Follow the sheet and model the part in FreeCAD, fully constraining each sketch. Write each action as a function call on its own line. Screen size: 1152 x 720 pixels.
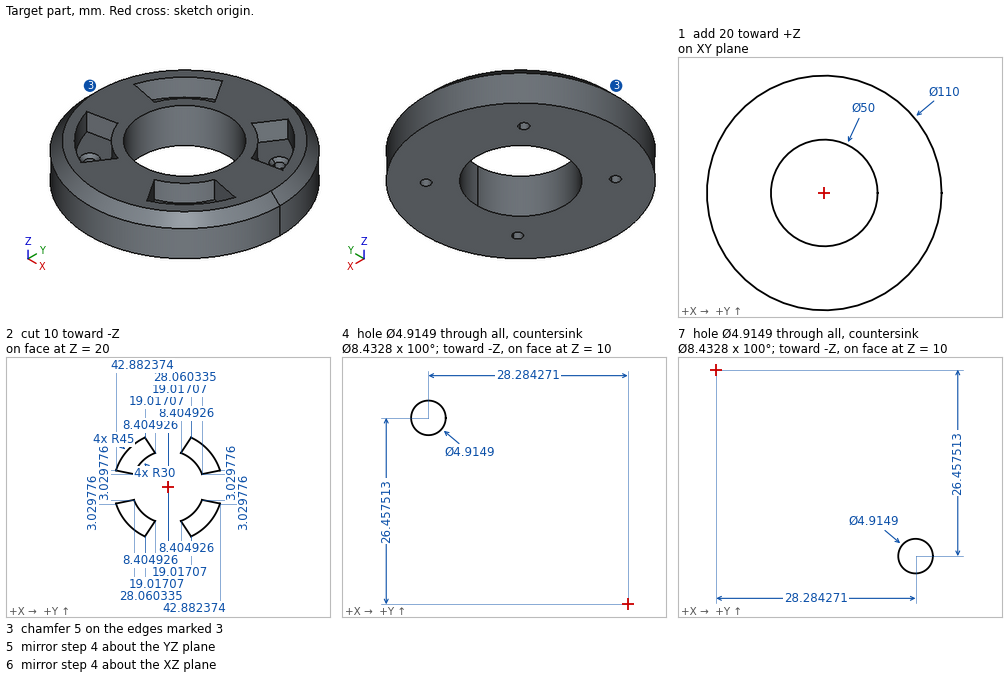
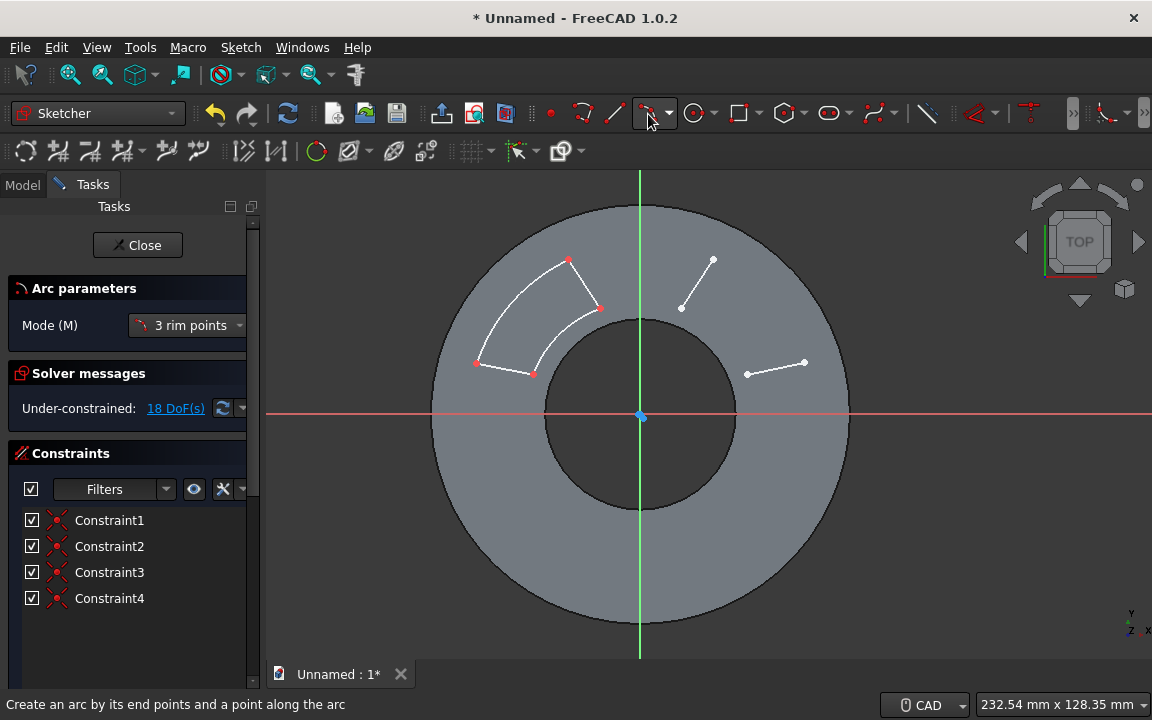
click(804, 363)
click(713, 260)
click(769, 301)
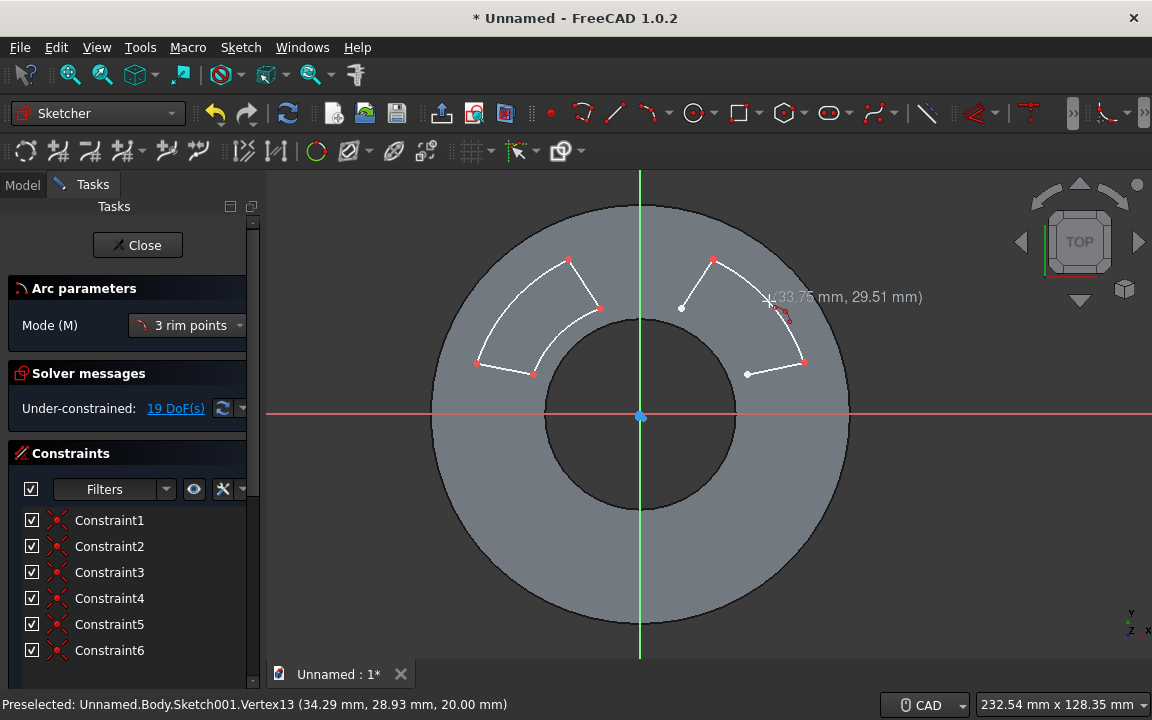
click(681, 309)
click(747, 375)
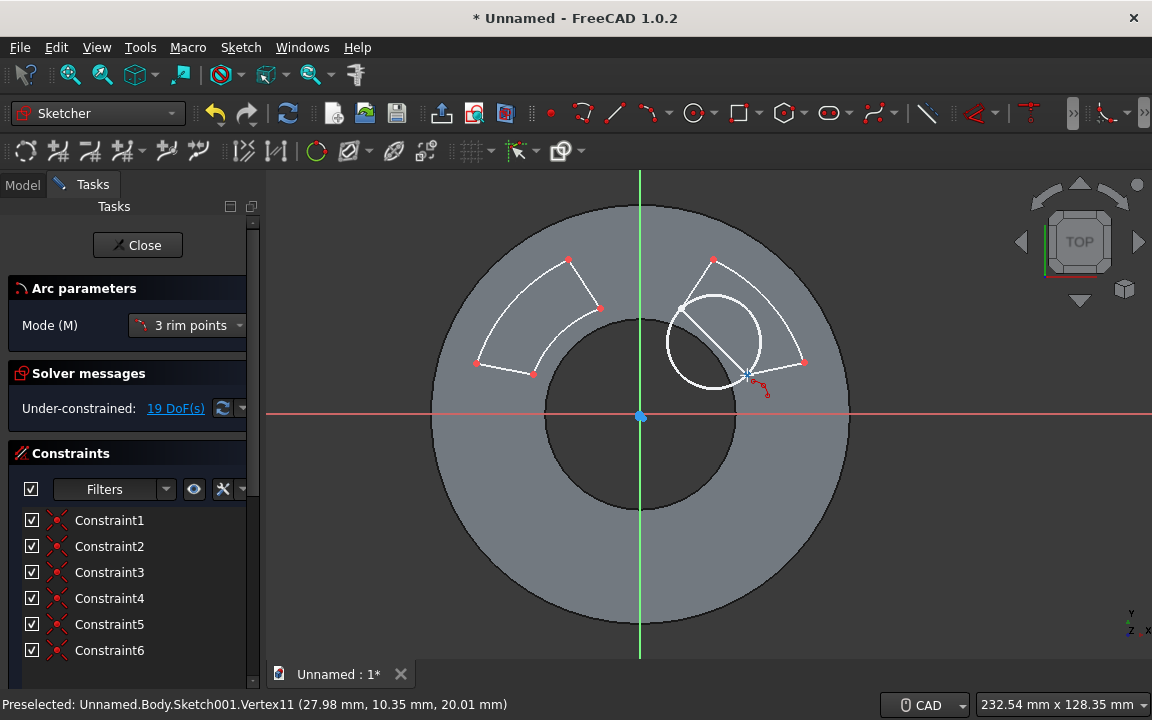
scroll(721, 334, up, 3)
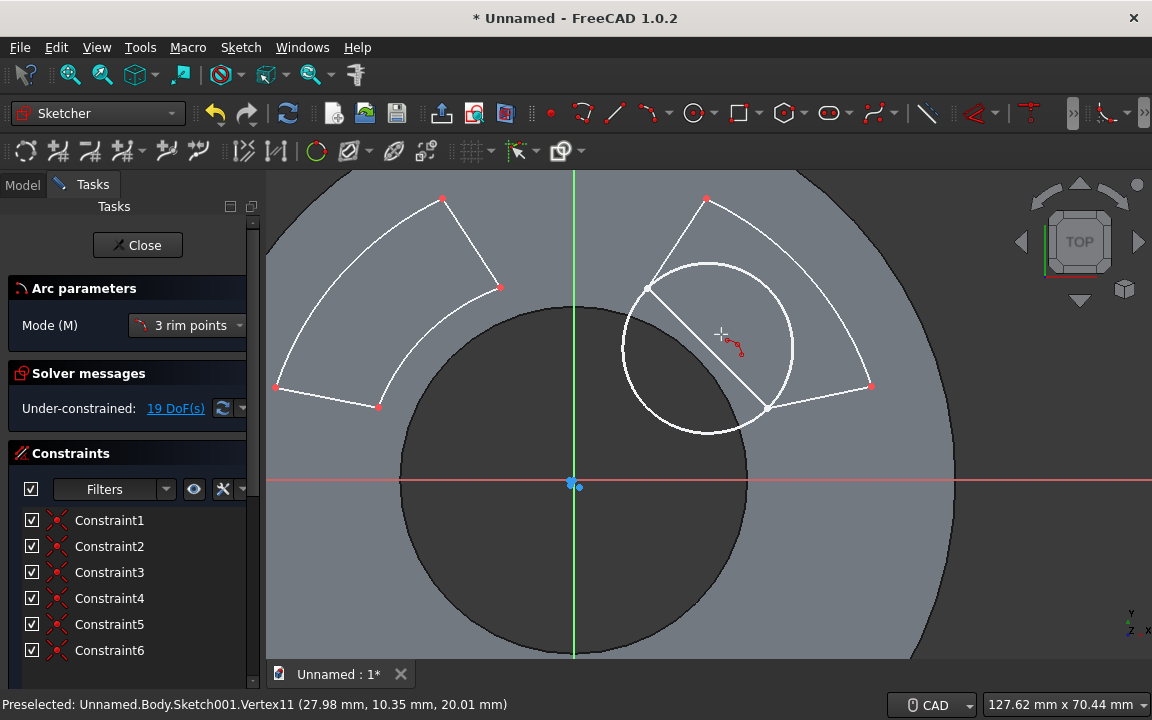
click(721, 333)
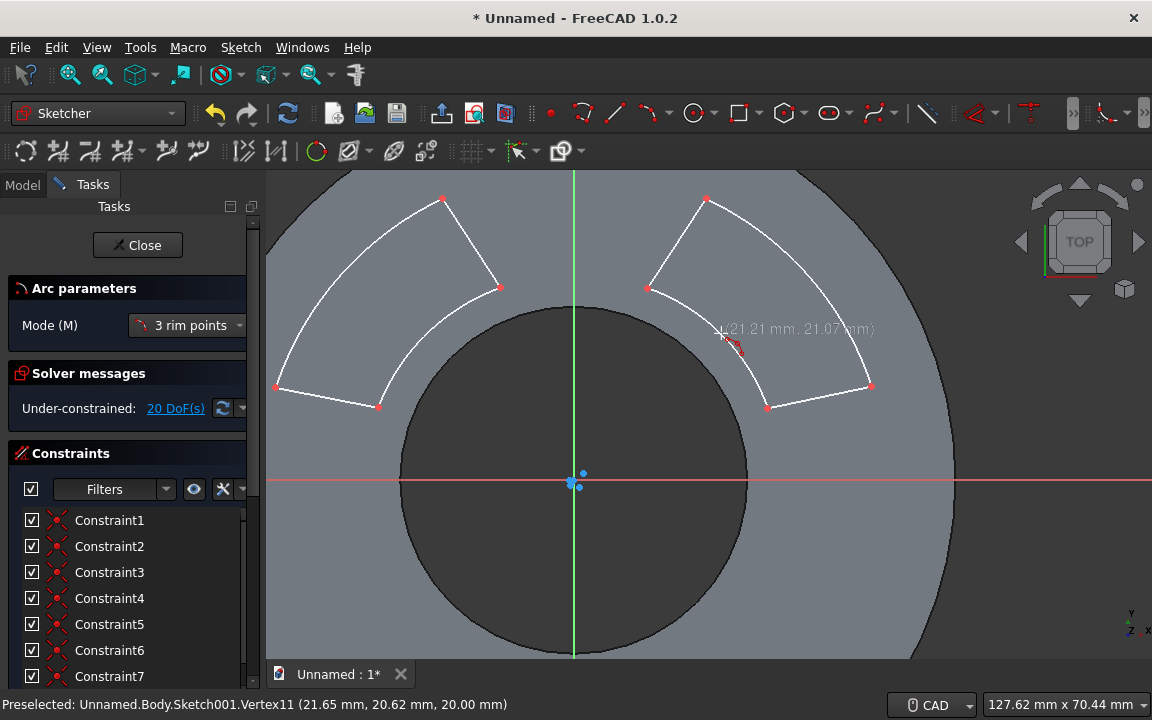
click(616, 114)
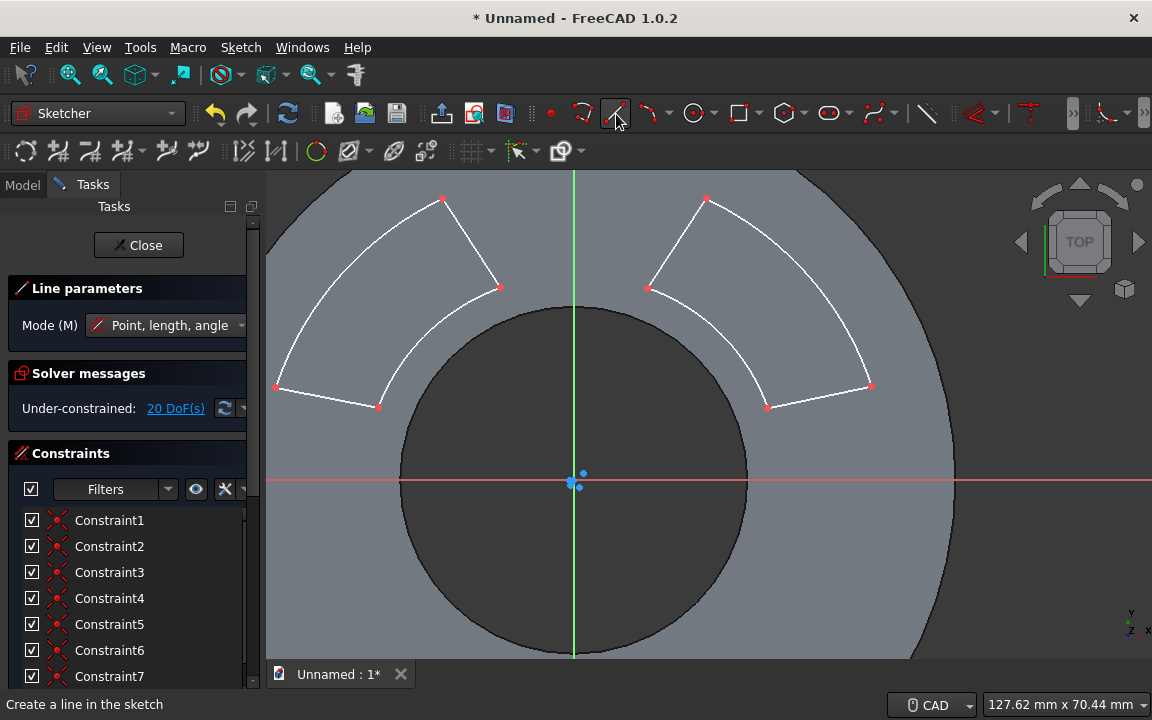
scroll(722, 335, down, 3)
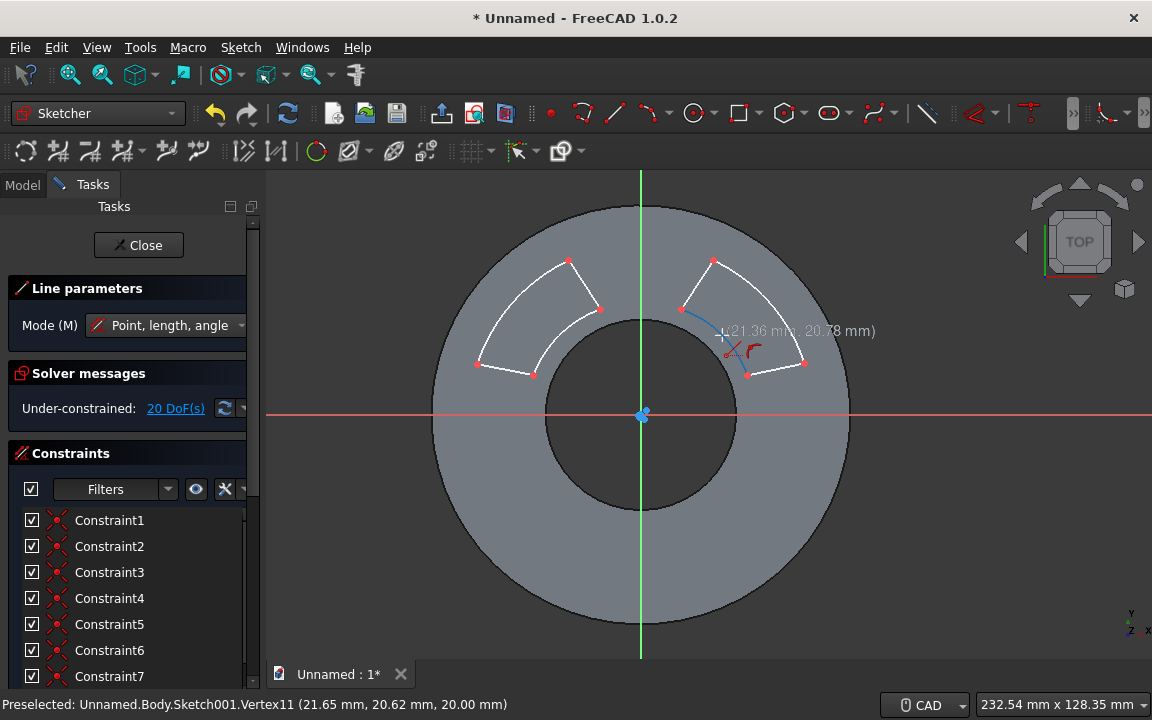
click(681, 522)
click(713, 570)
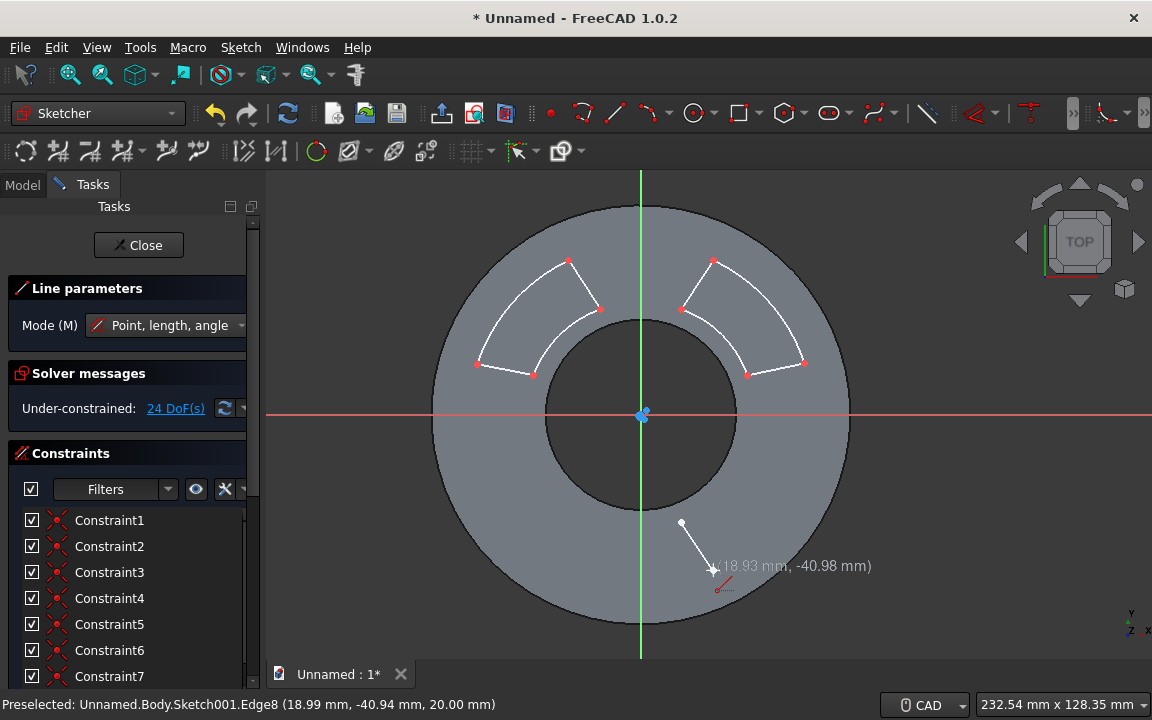
click(804, 467)
click(748, 455)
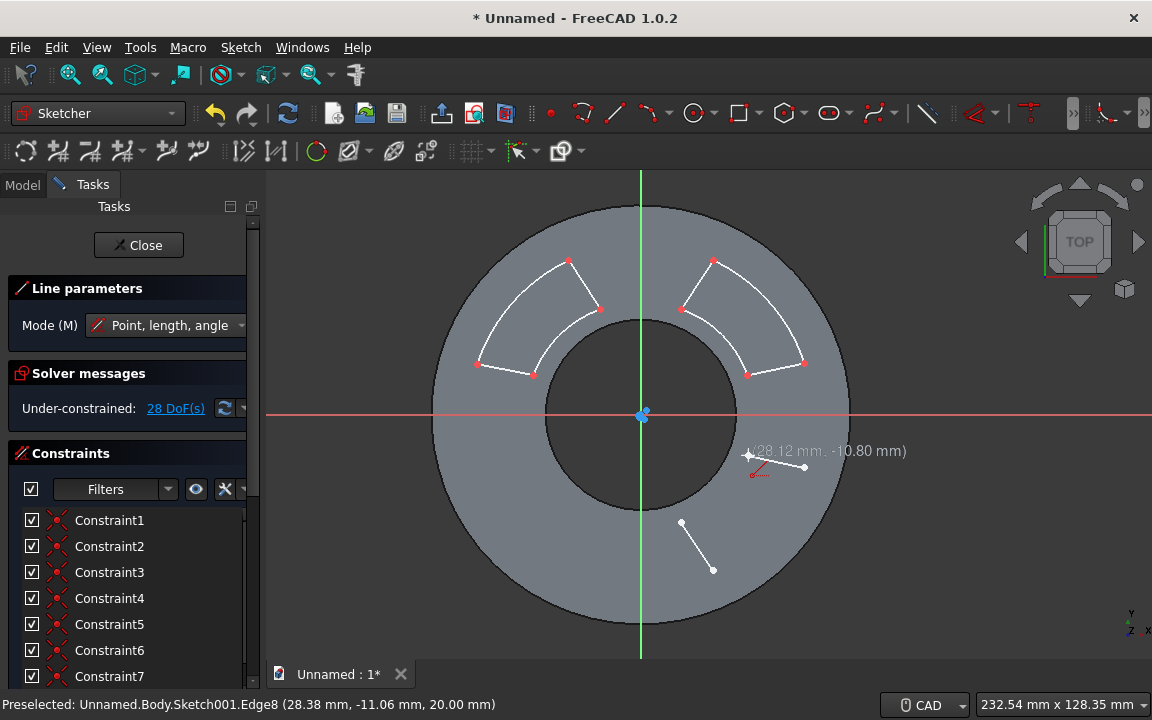
click(648, 114)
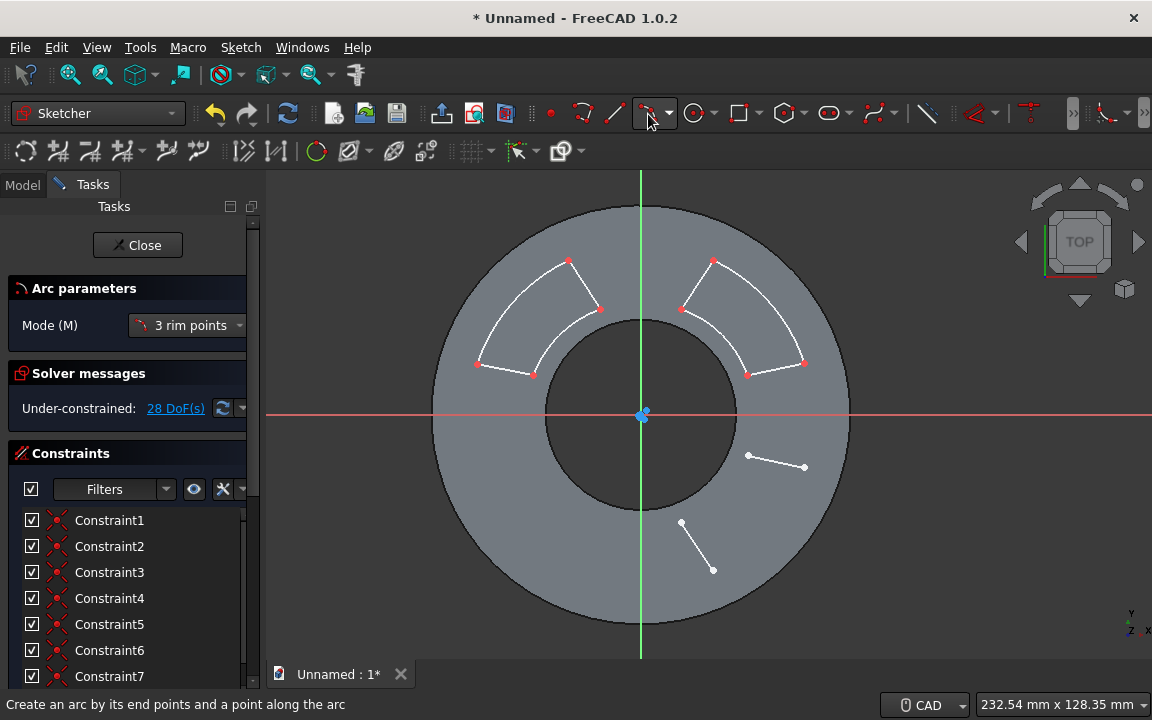
click(713, 571)
click(804, 468)
click(770, 528)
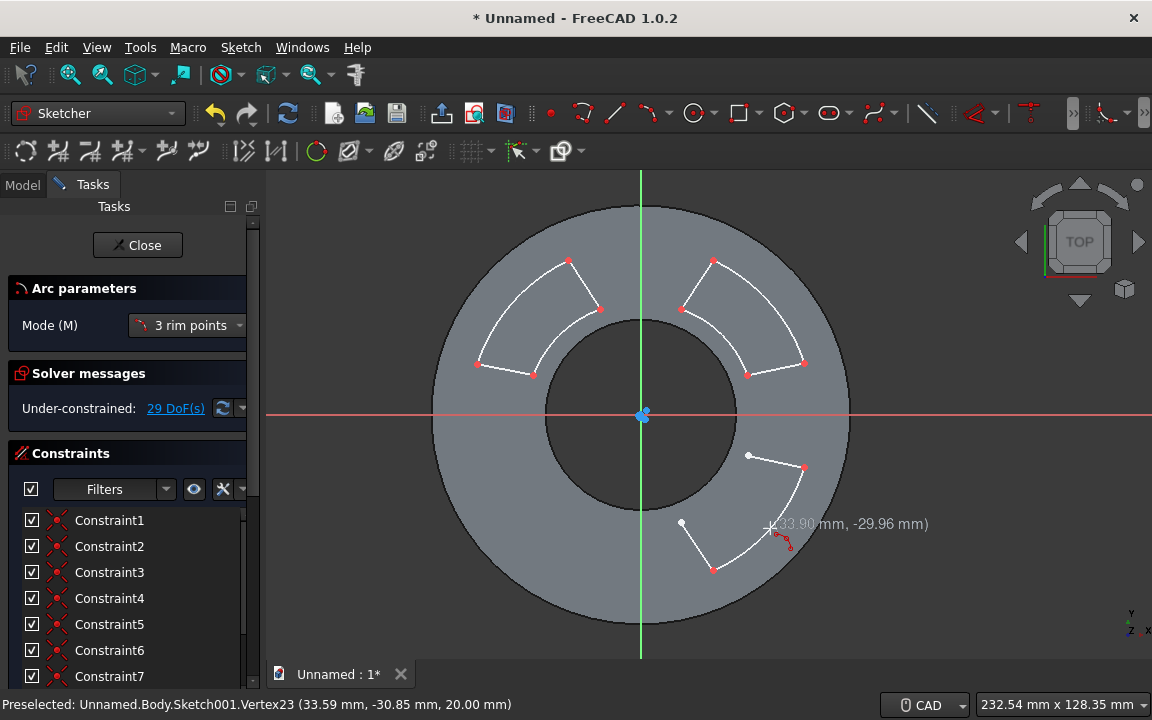
click(748, 456)
click(681, 523)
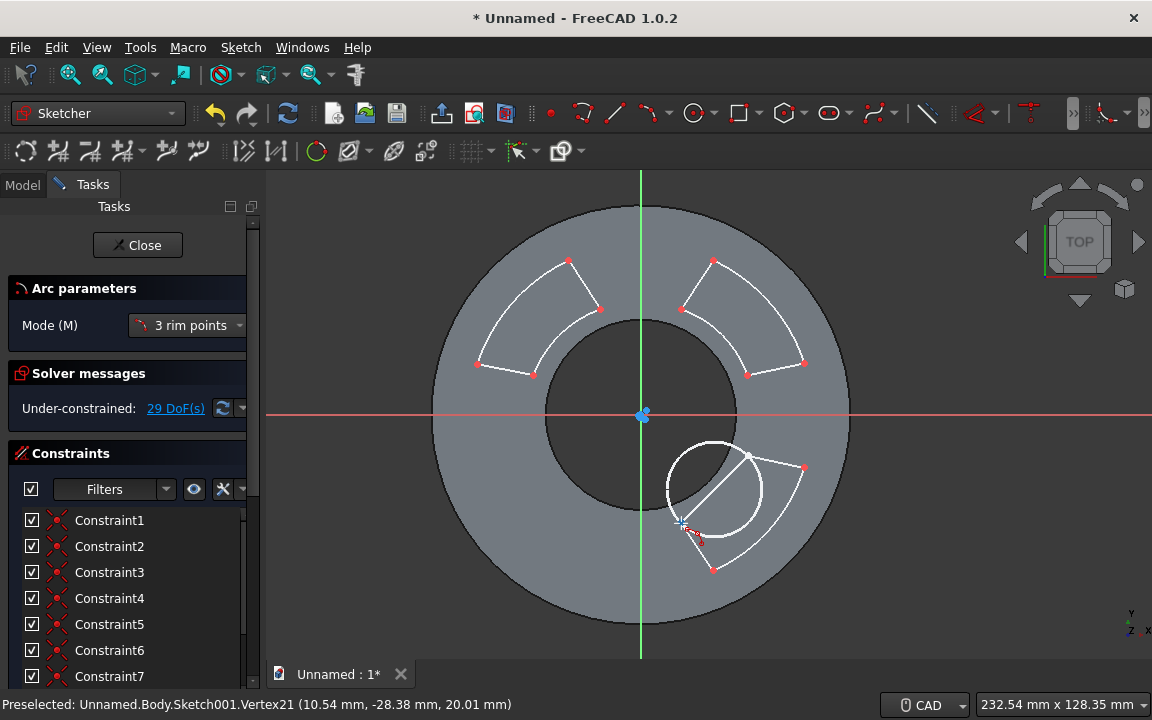
scroll(722, 496, up, 3)